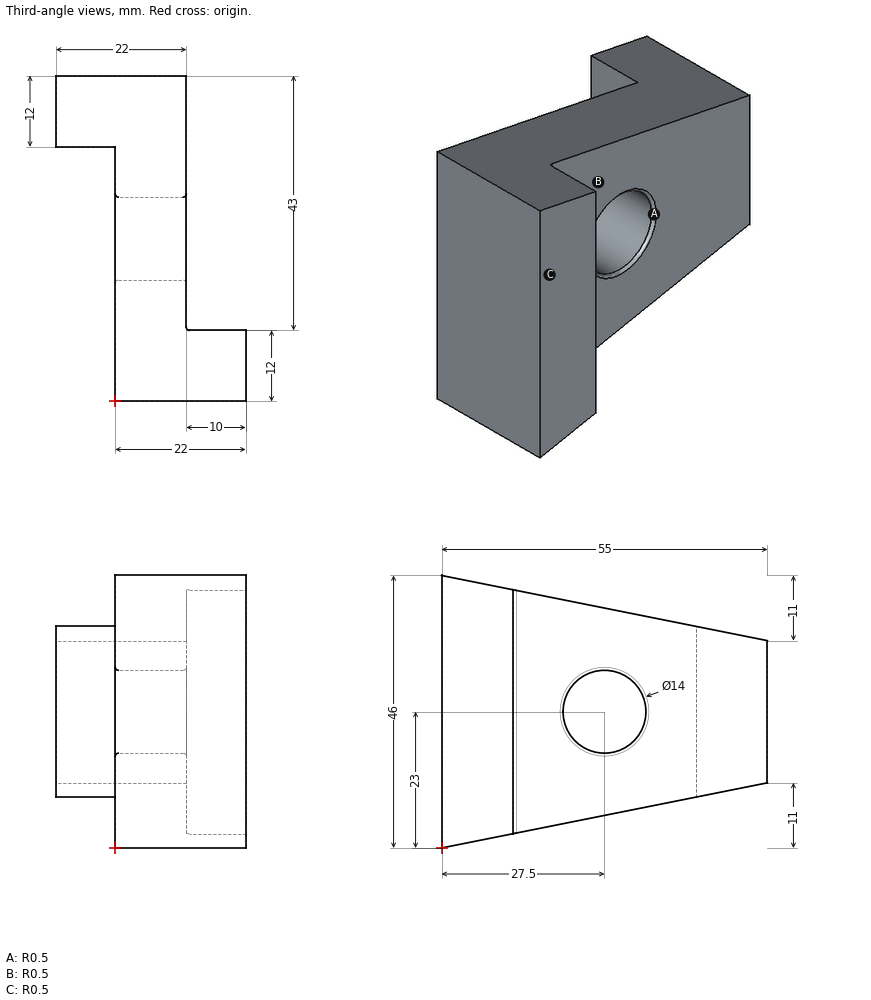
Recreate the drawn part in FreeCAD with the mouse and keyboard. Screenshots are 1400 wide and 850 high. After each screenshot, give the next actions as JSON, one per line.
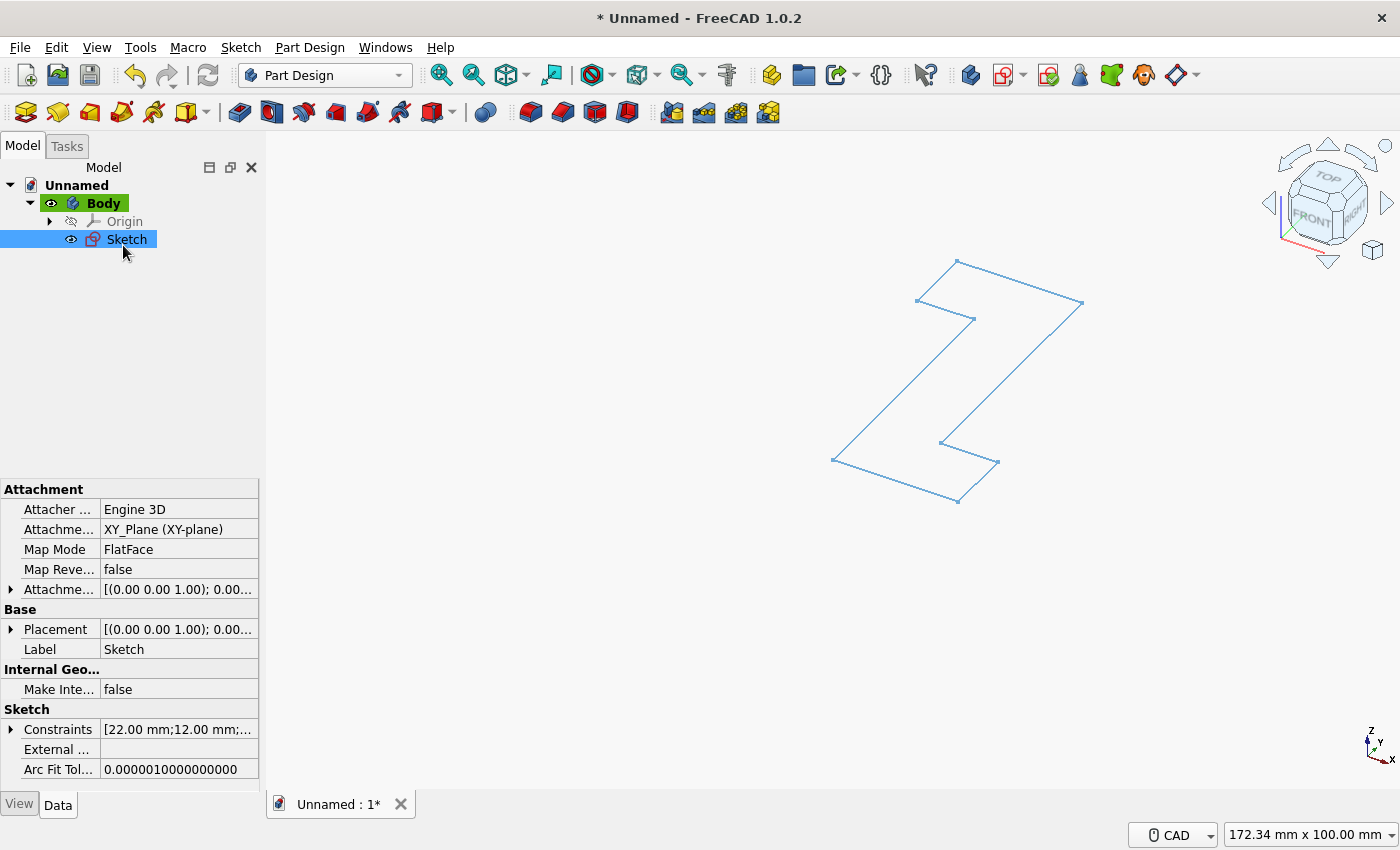
{"action": "left_click", "coordinate": [26, 112]}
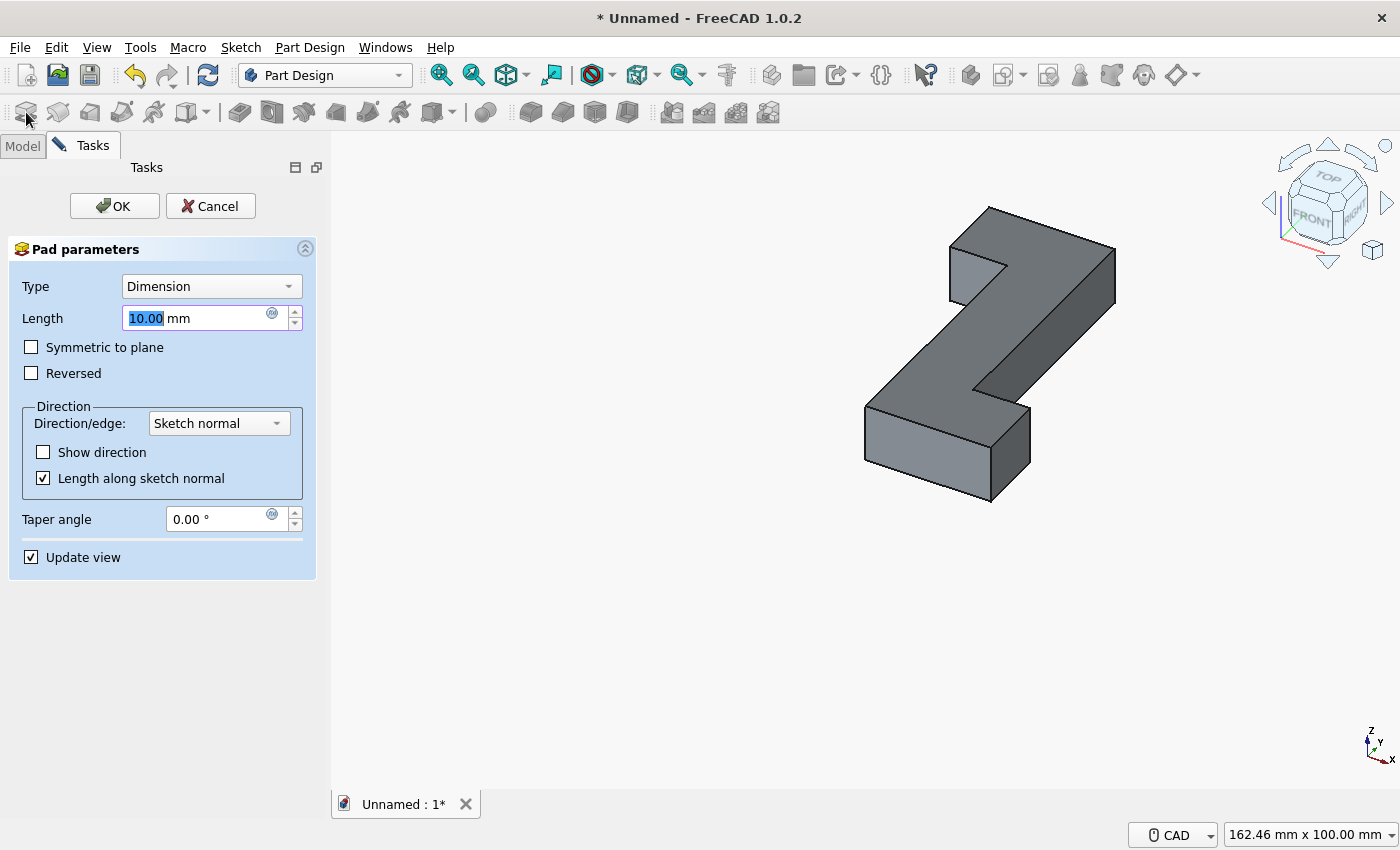
{"action": "type", "text": "46"}
{"action": "key", "text": "Tab"}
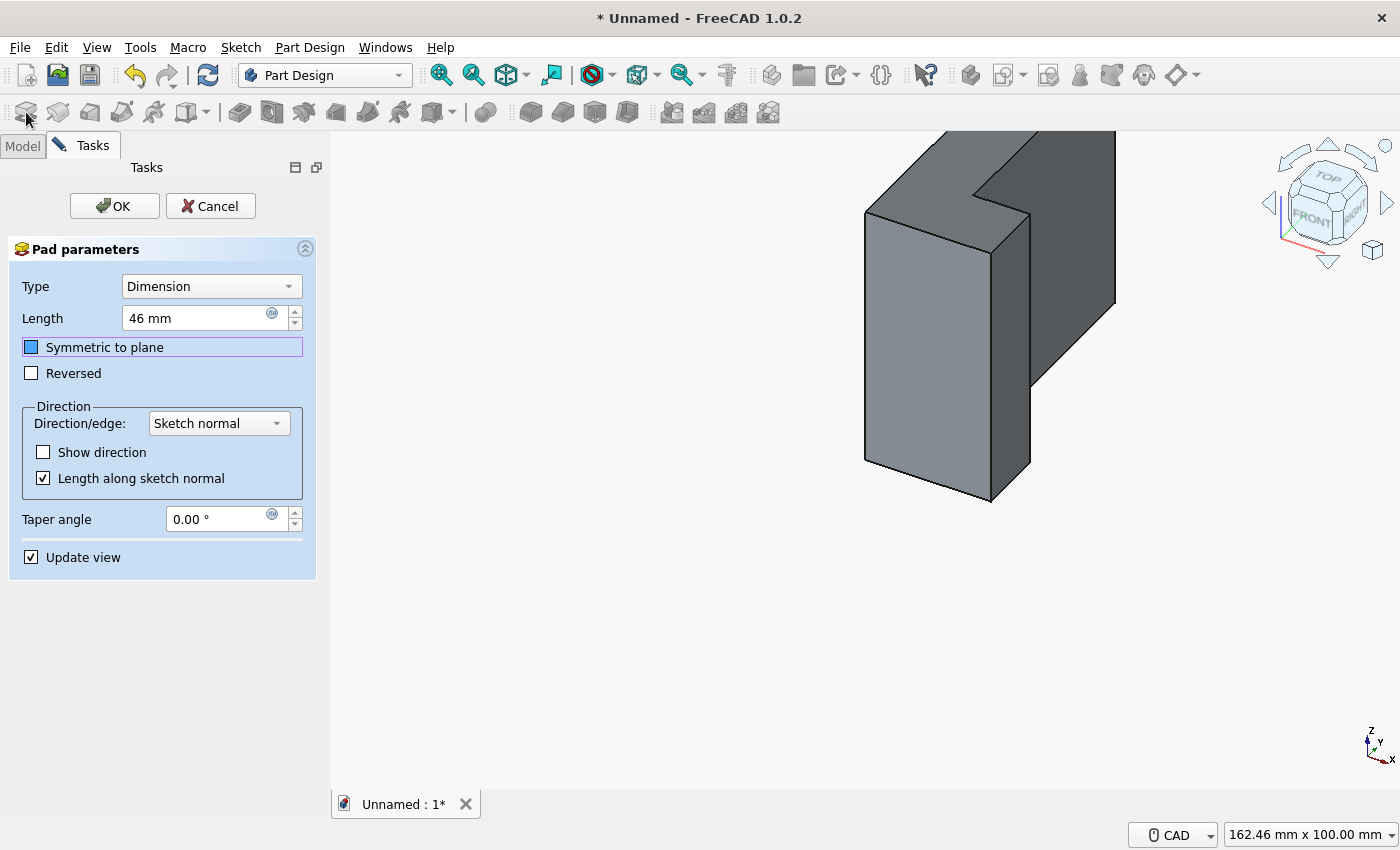
{"action": "left_click", "coordinate": [115, 206]}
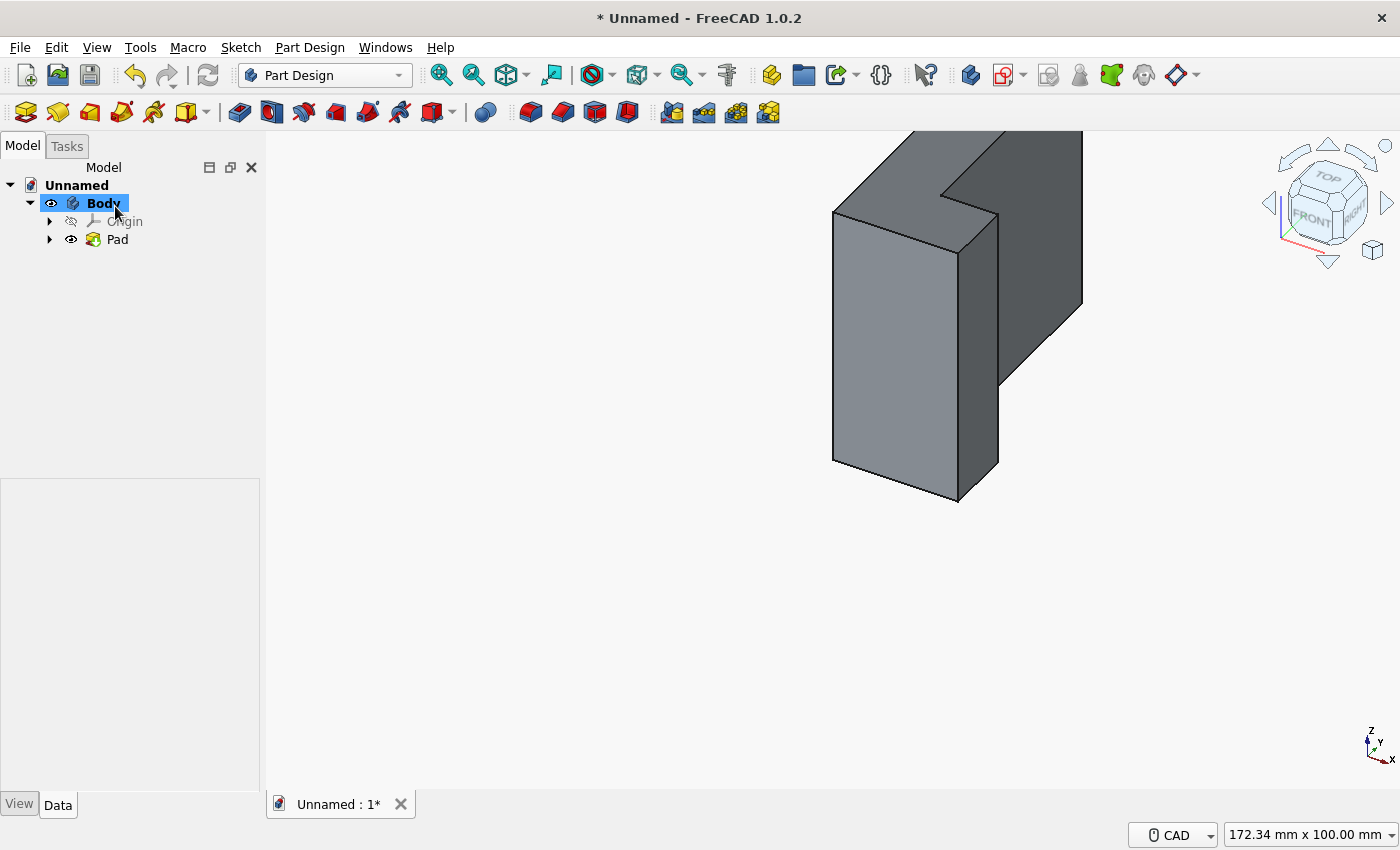
{"action": "left_click", "coordinate": [442, 76]}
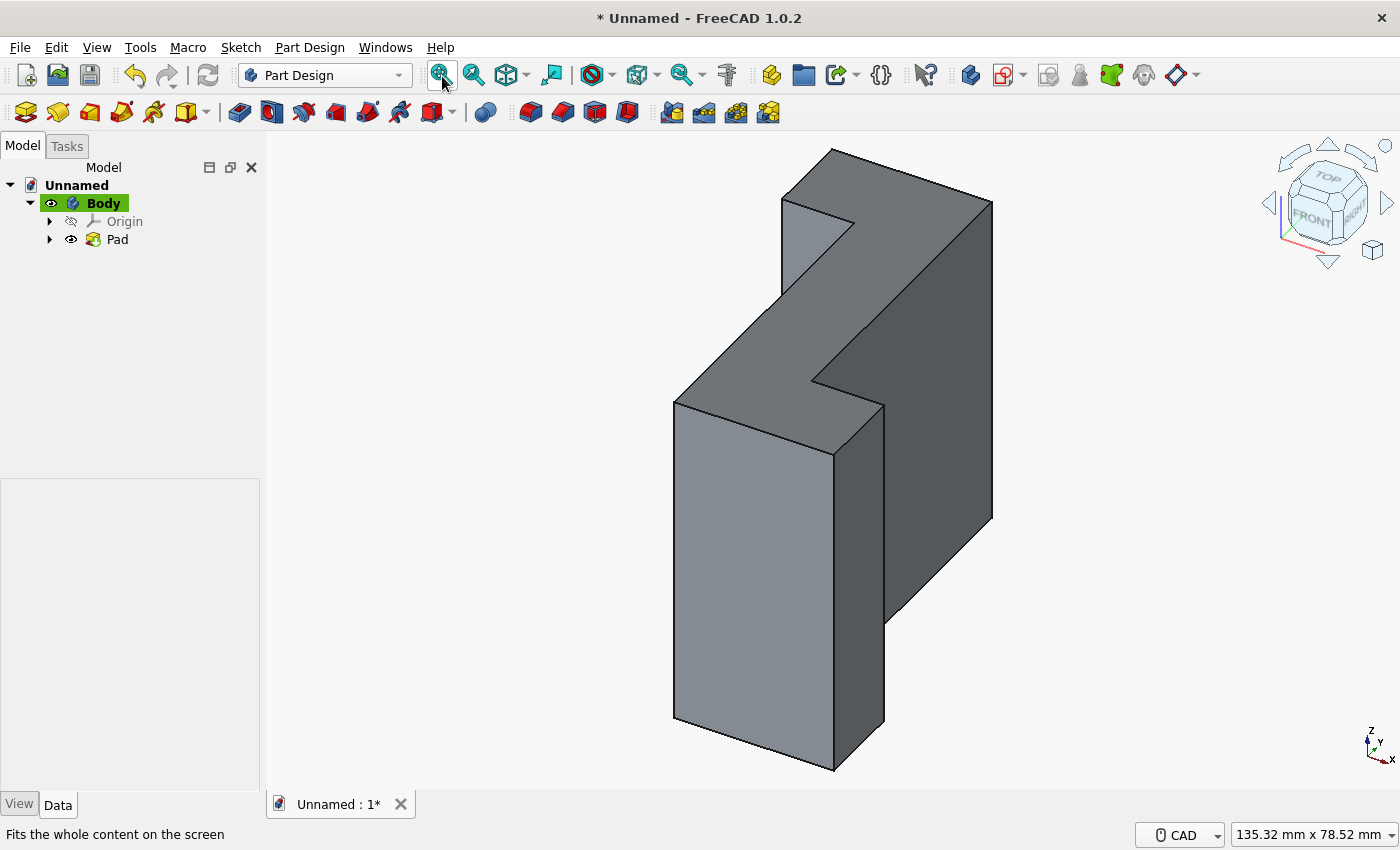
{"action": "left_click", "coordinate": [859, 497]}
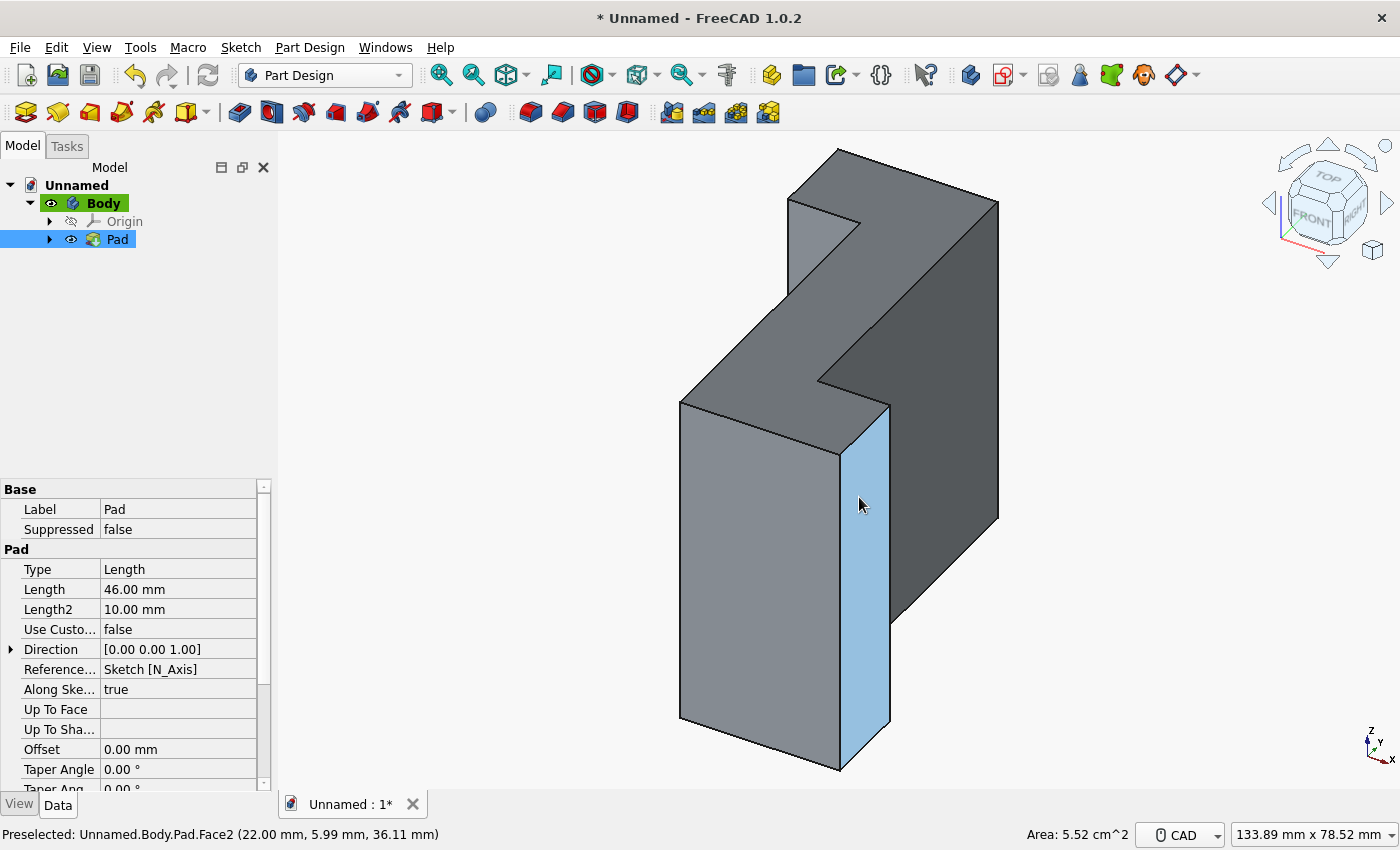
{"action": "left_click", "coordinate": [1004, 76]}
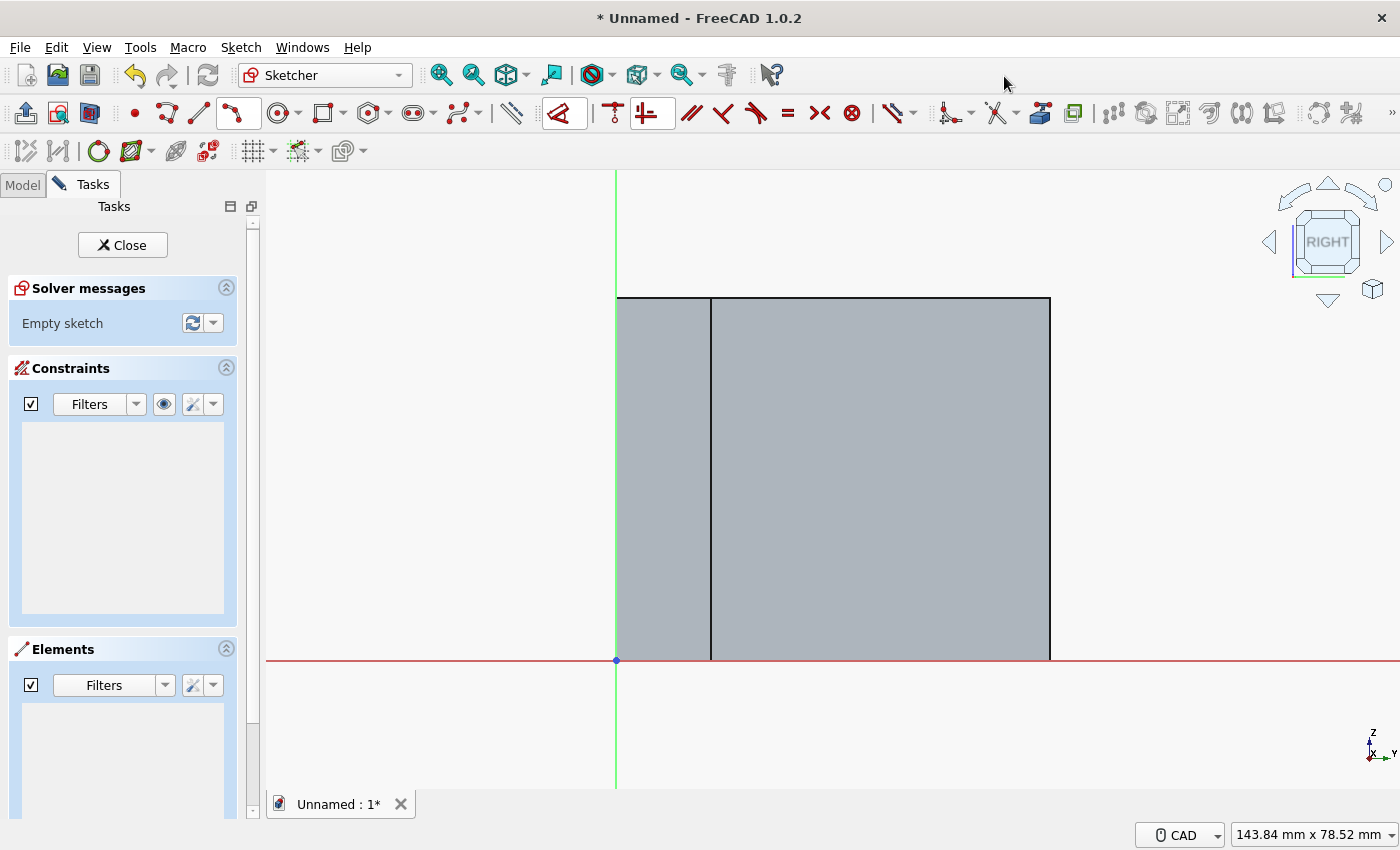
{"action": "left_click", "coordinate": [168, 114]}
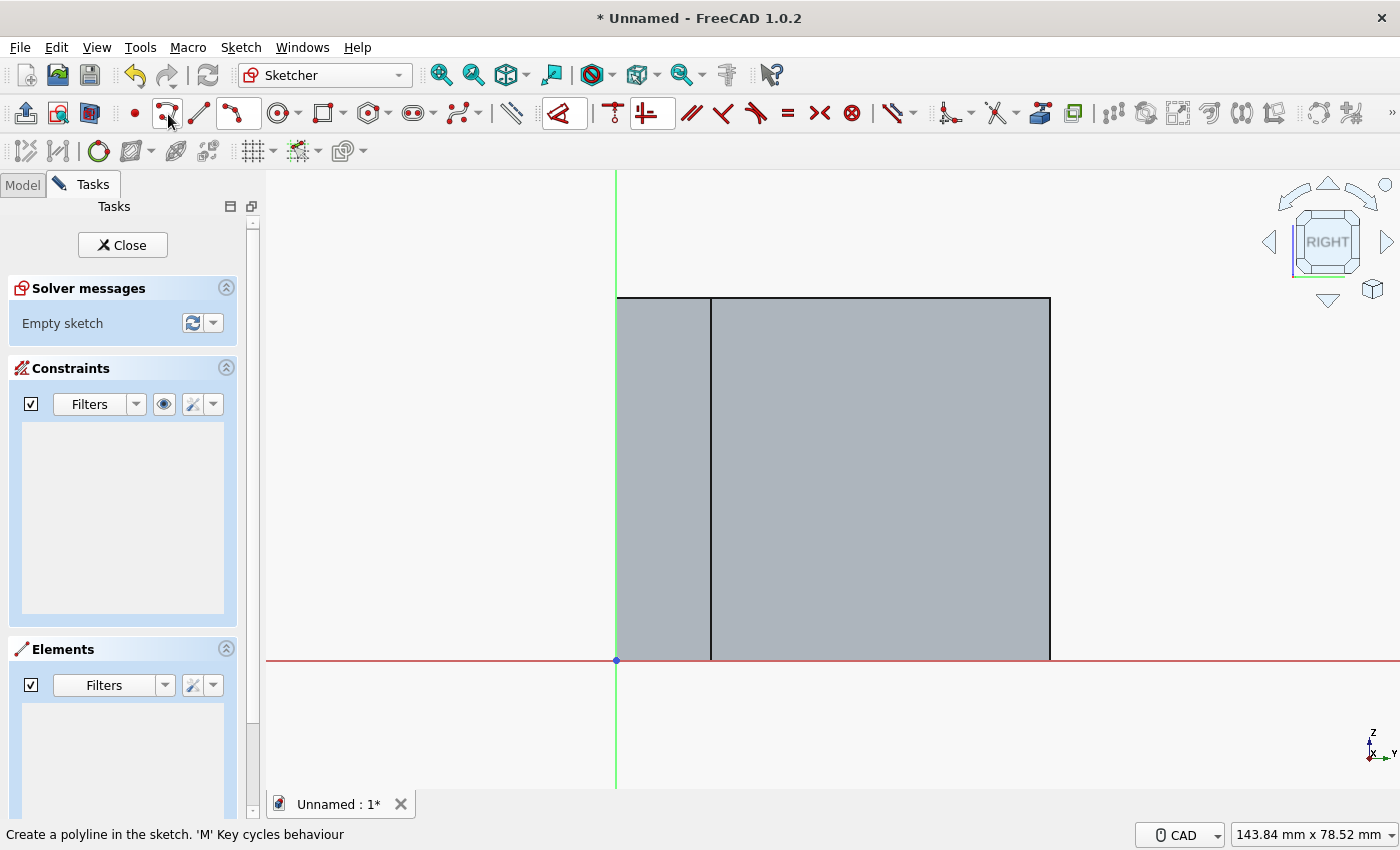
{"action": "left_click", "coordinate": [616, 298]}
{"action": "left_click", "coordinate": [1050, 385]}
{"action": "left_click", "coordinate": [1050, 298]}
{"action": "left_click", "coordinate": [616, 299]}